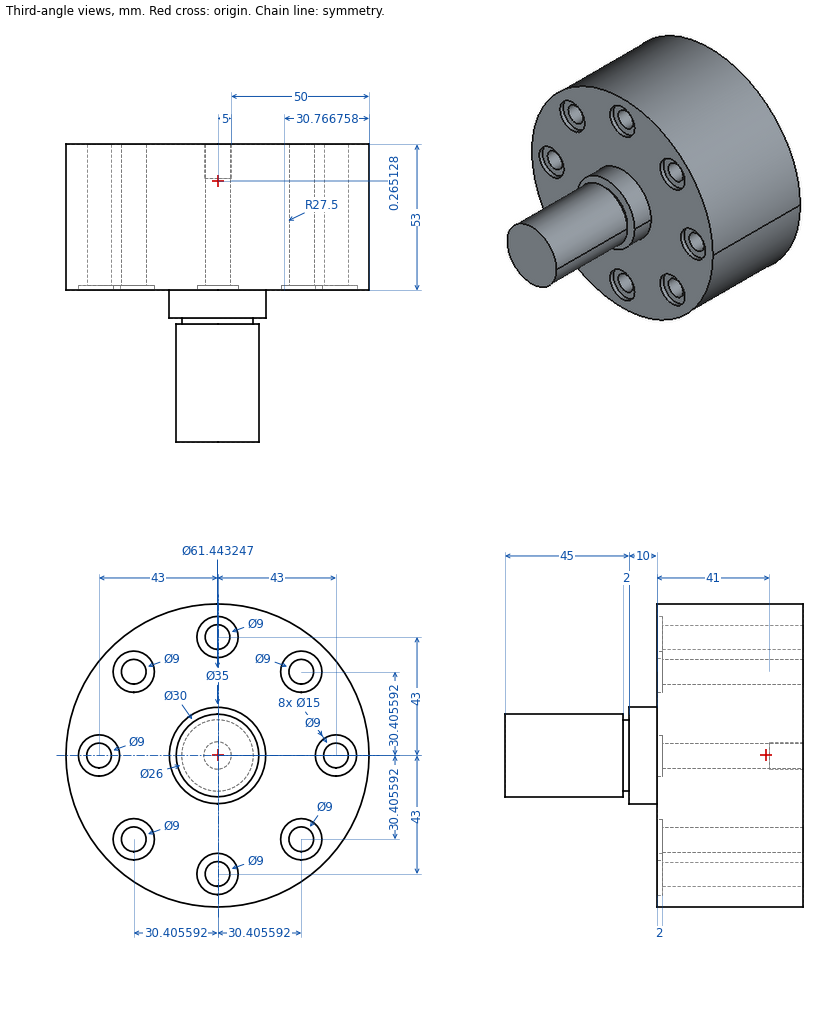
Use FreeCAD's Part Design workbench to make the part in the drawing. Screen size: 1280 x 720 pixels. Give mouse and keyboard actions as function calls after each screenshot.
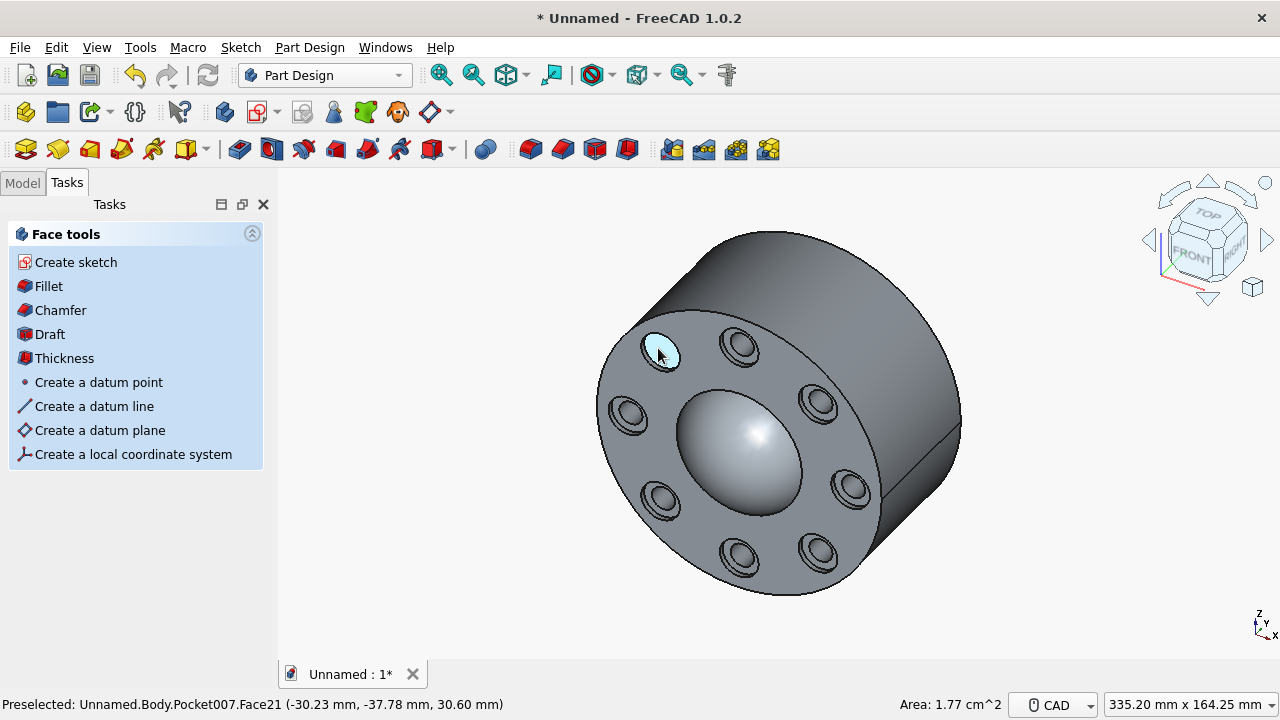
click(258, 112)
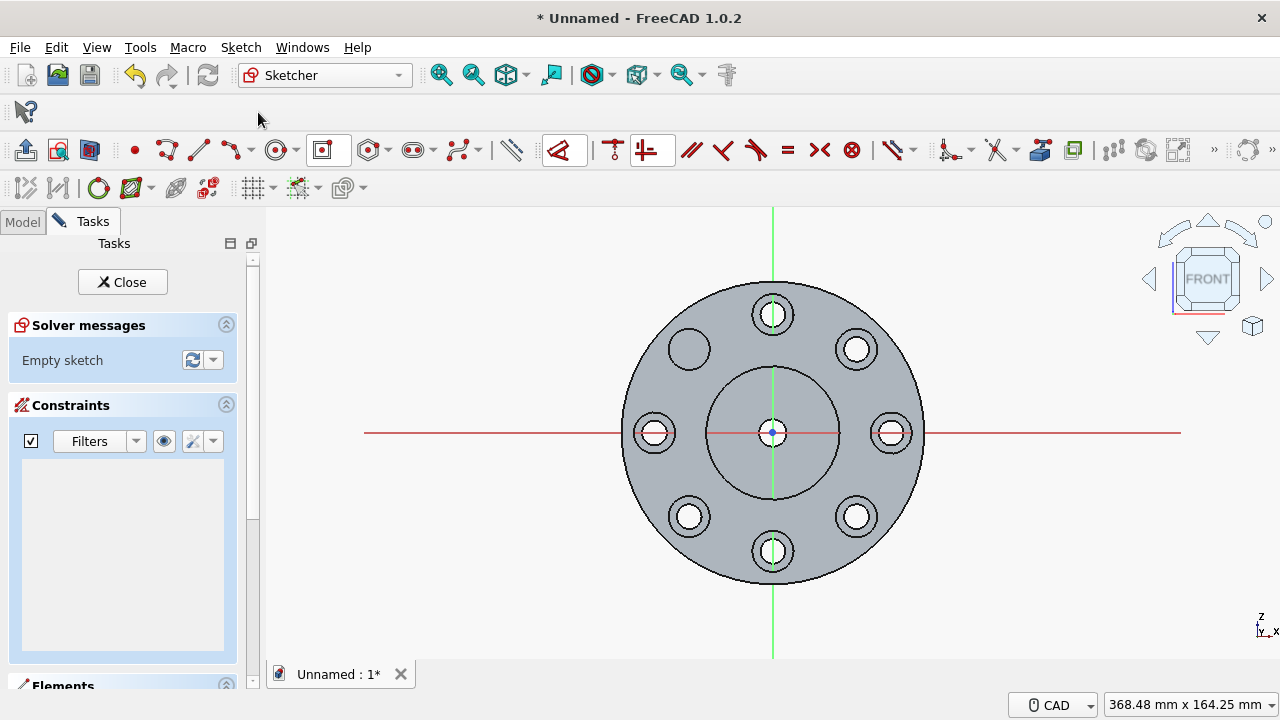
click(90, 150)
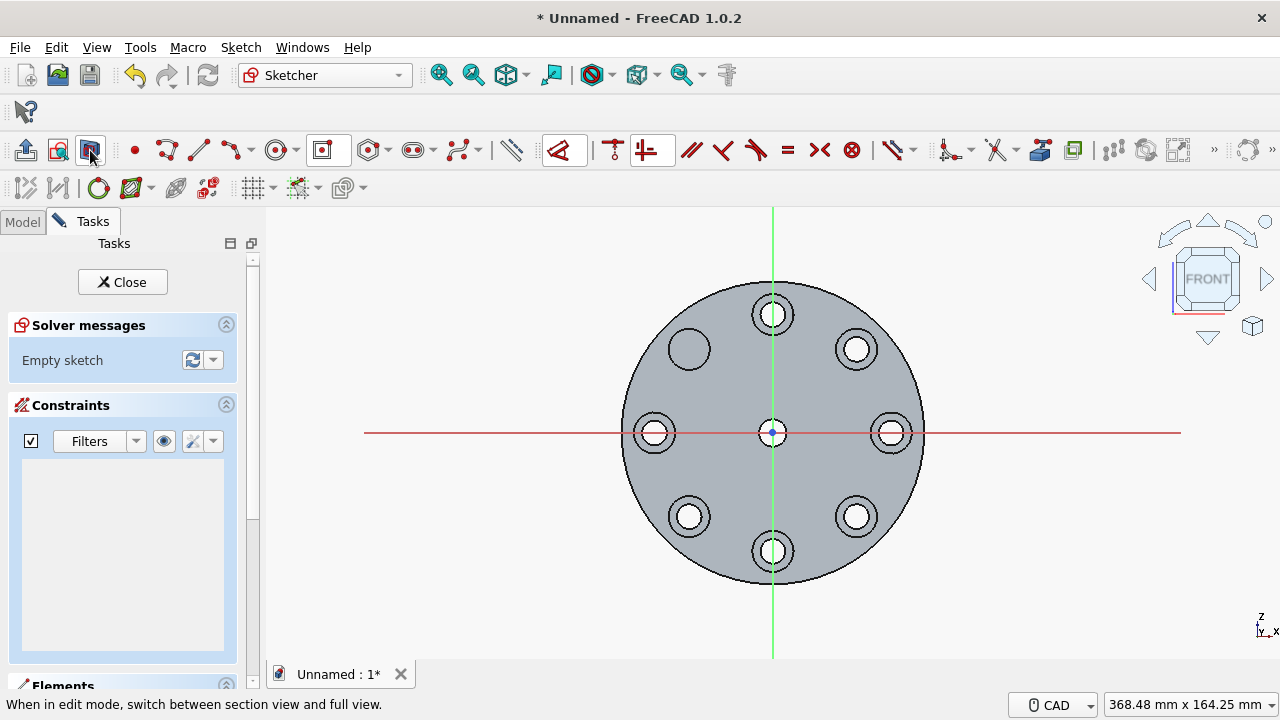
scroll(688, 341, up, 12)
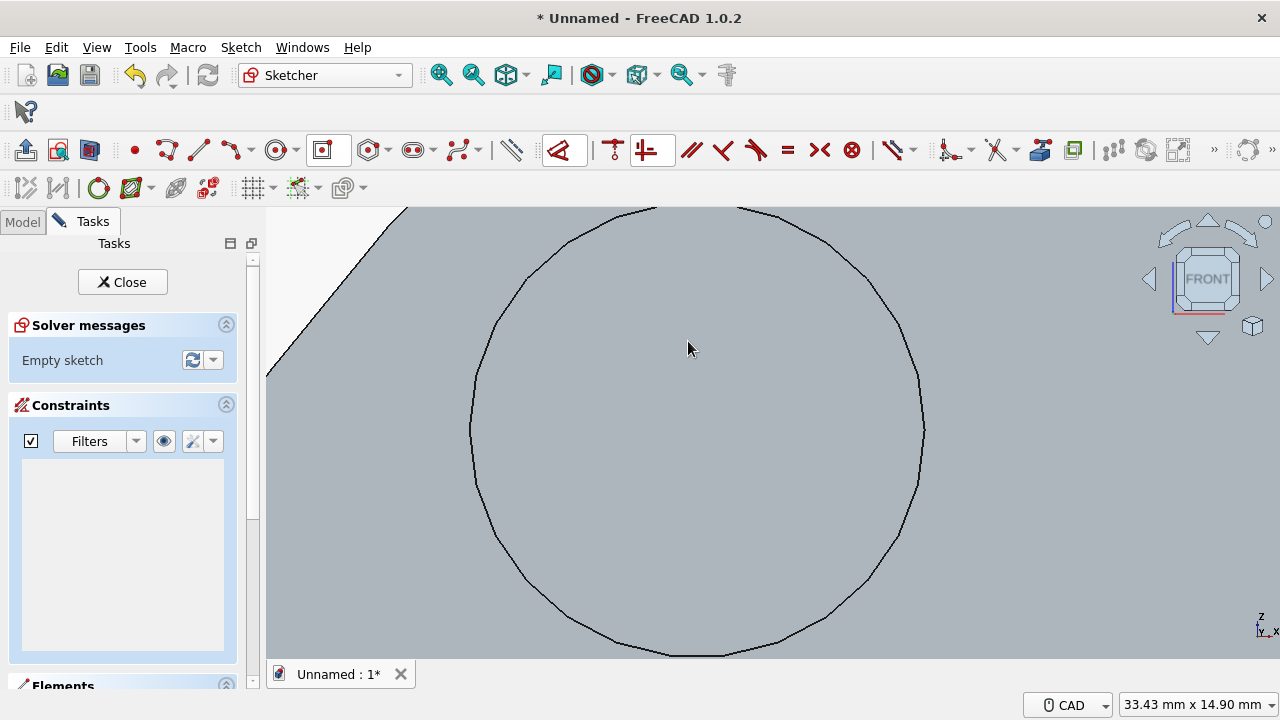
click(276, 150)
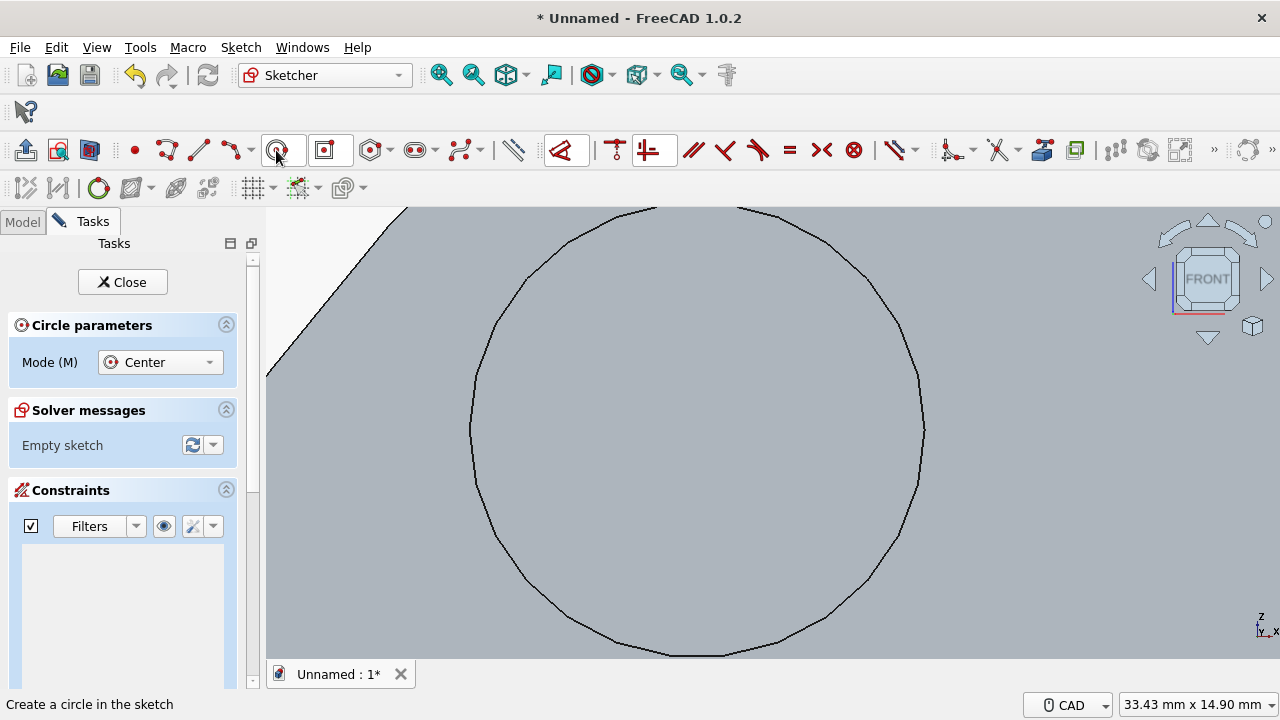
click(697, 430)
move(794, 333)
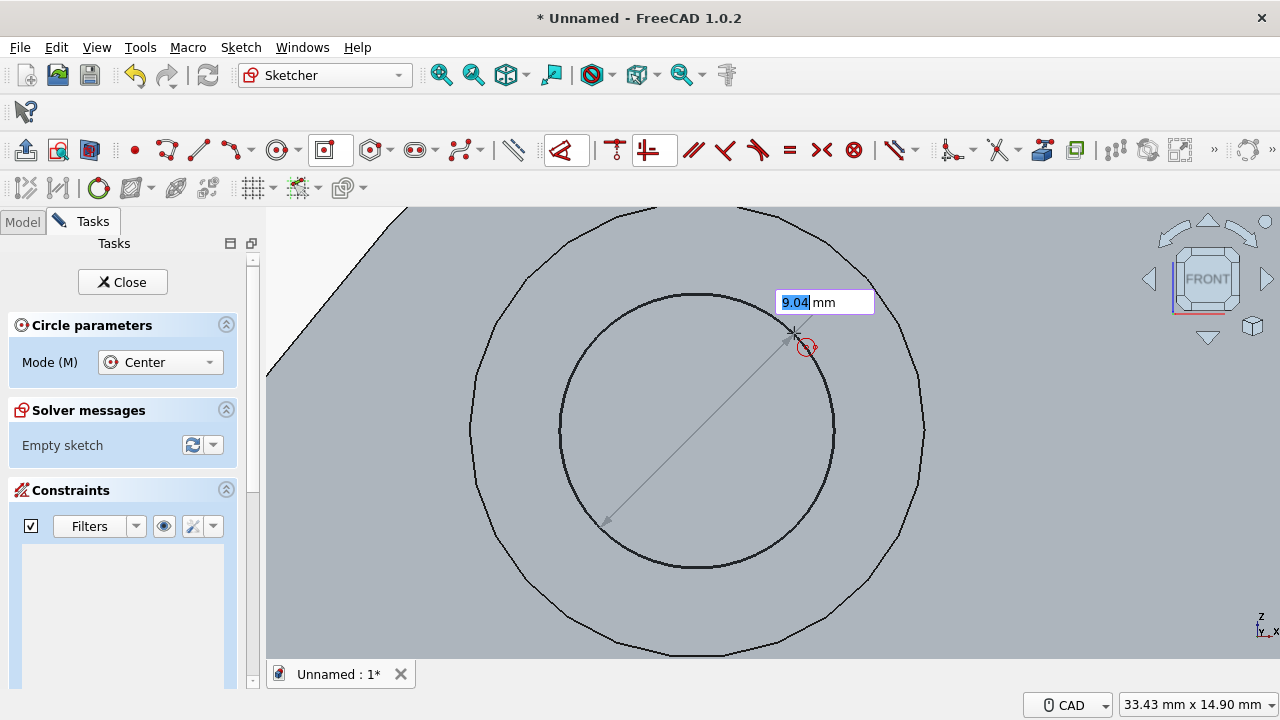
text(9)
key(Return)
key(Escape)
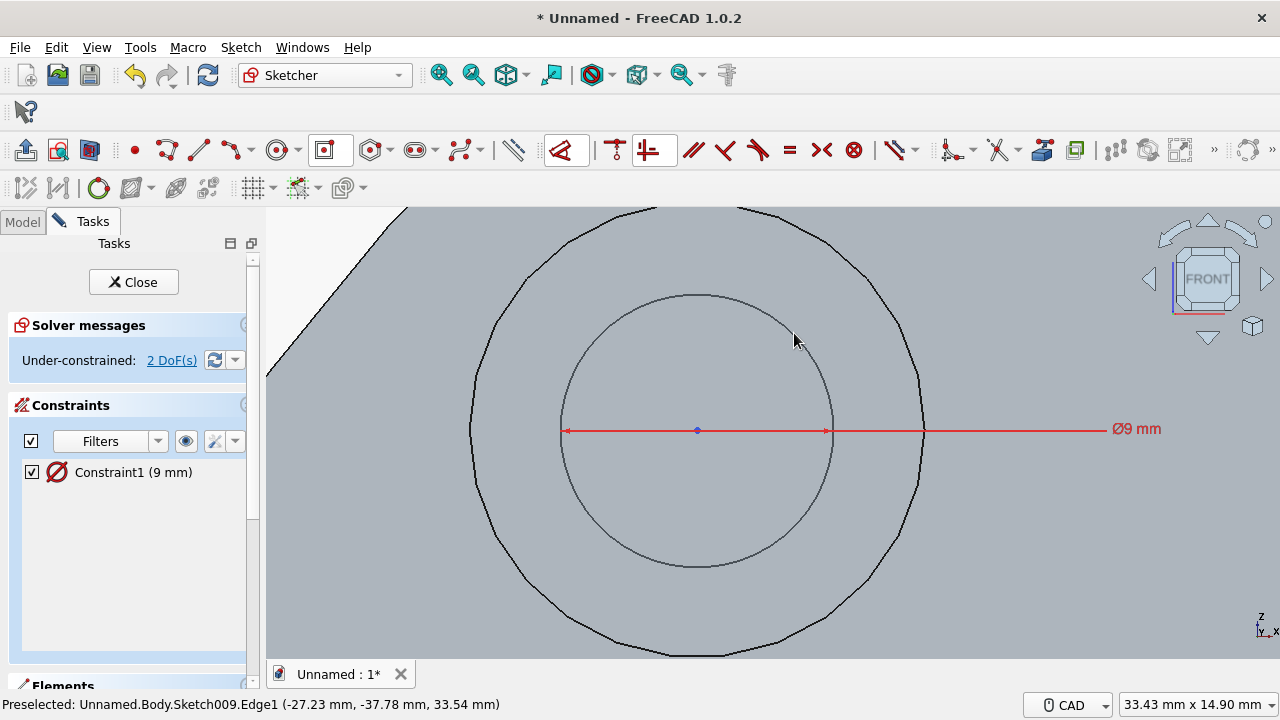
click(697, 431)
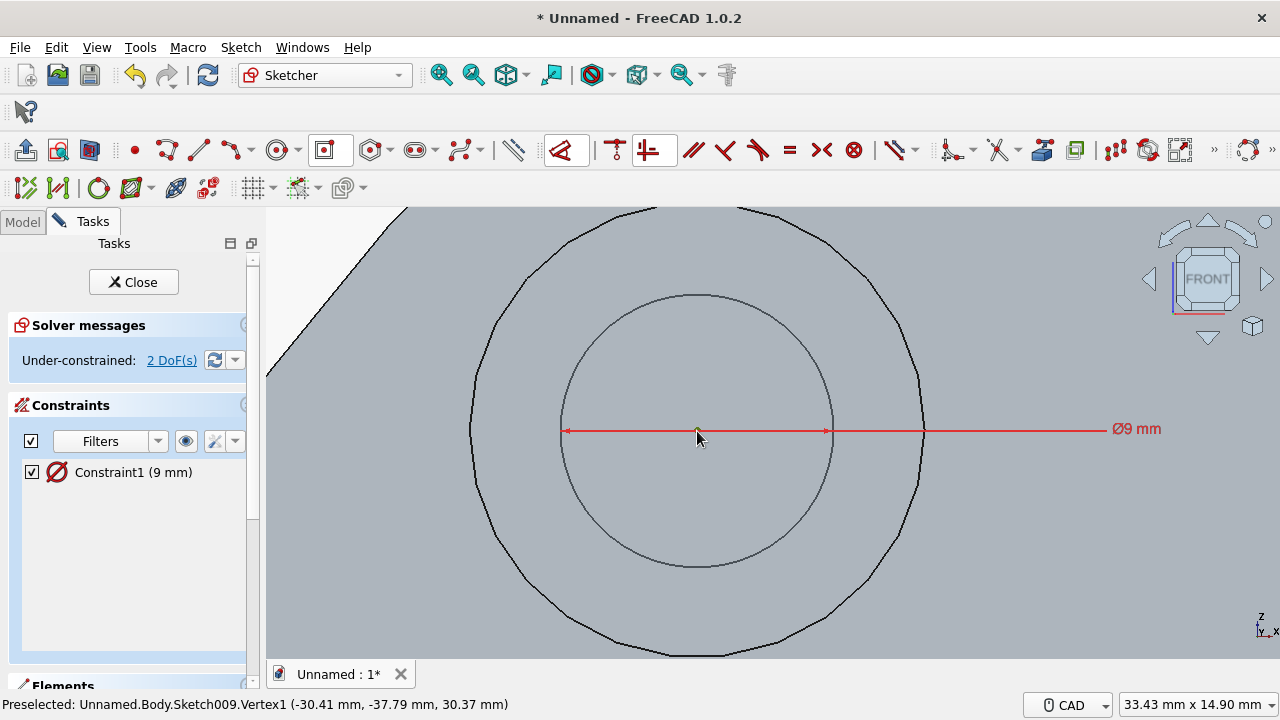
click(584, 150)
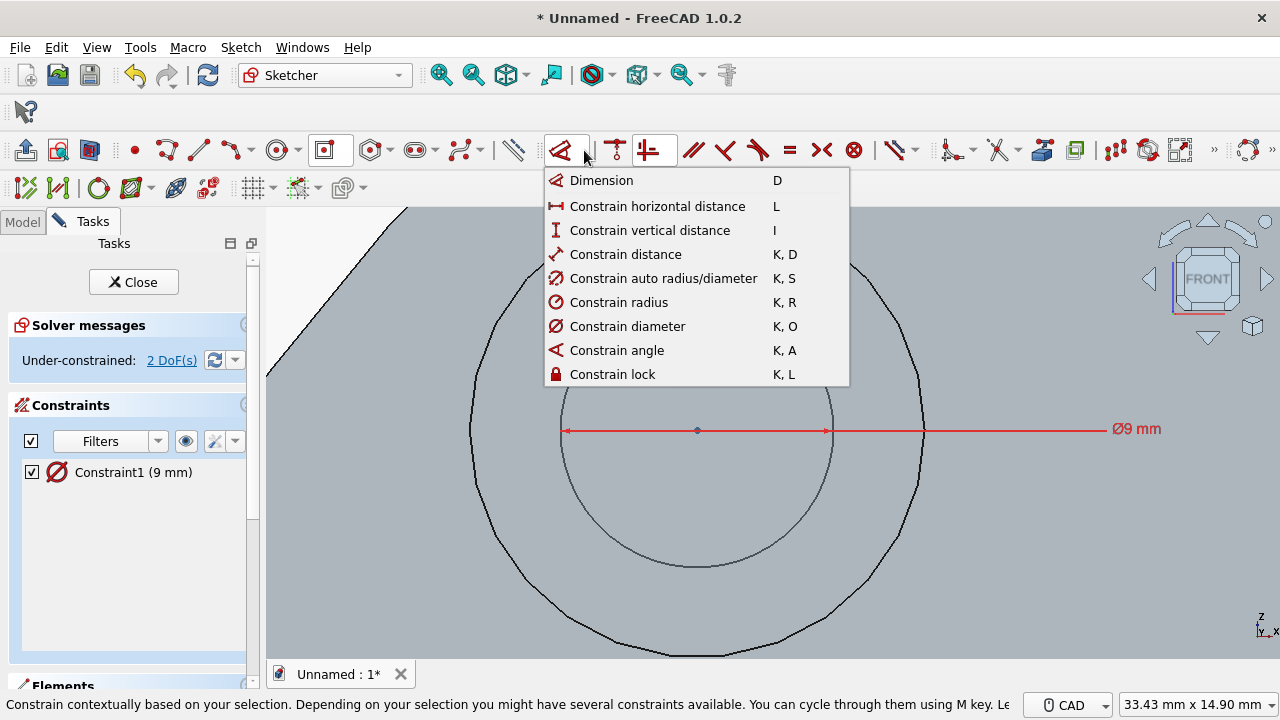
click(697, 206)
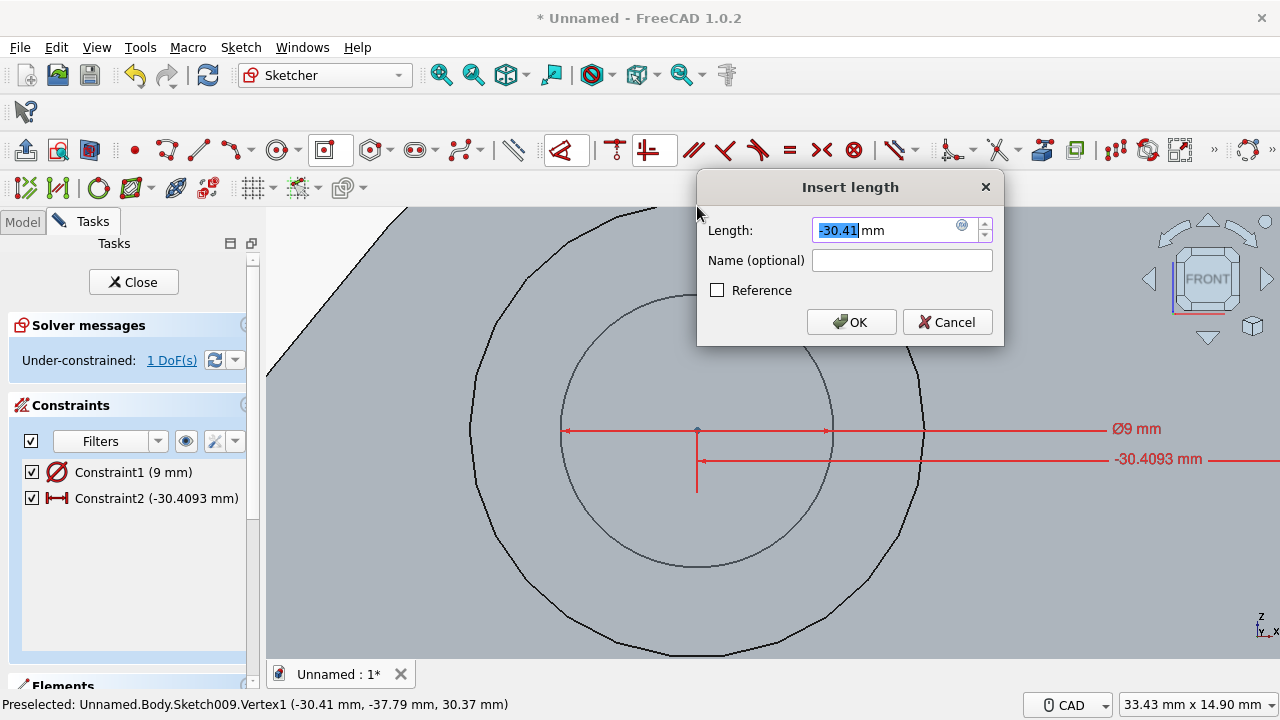
text(-30.405592)
key(Return)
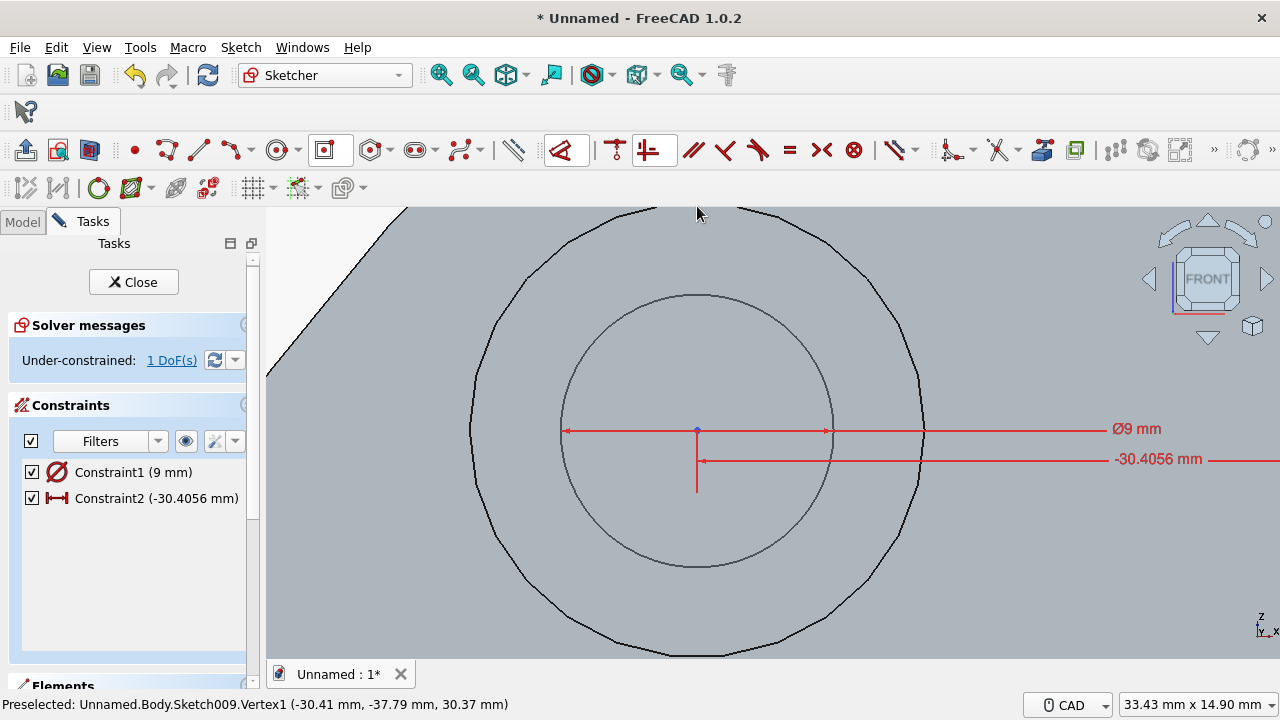
click(697, 431)